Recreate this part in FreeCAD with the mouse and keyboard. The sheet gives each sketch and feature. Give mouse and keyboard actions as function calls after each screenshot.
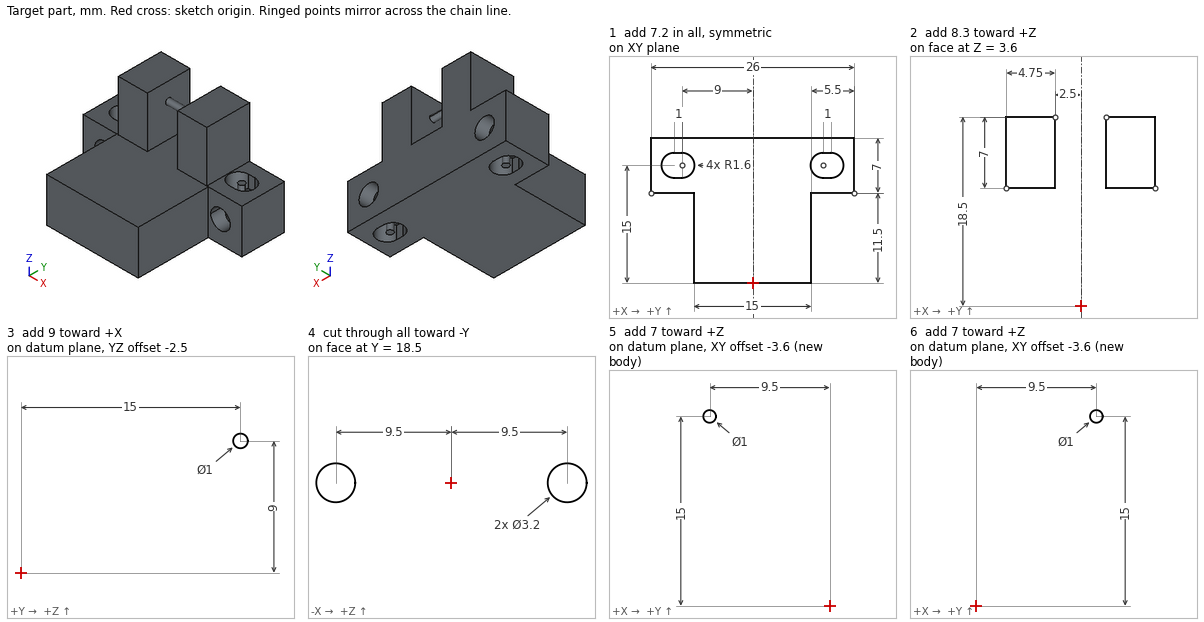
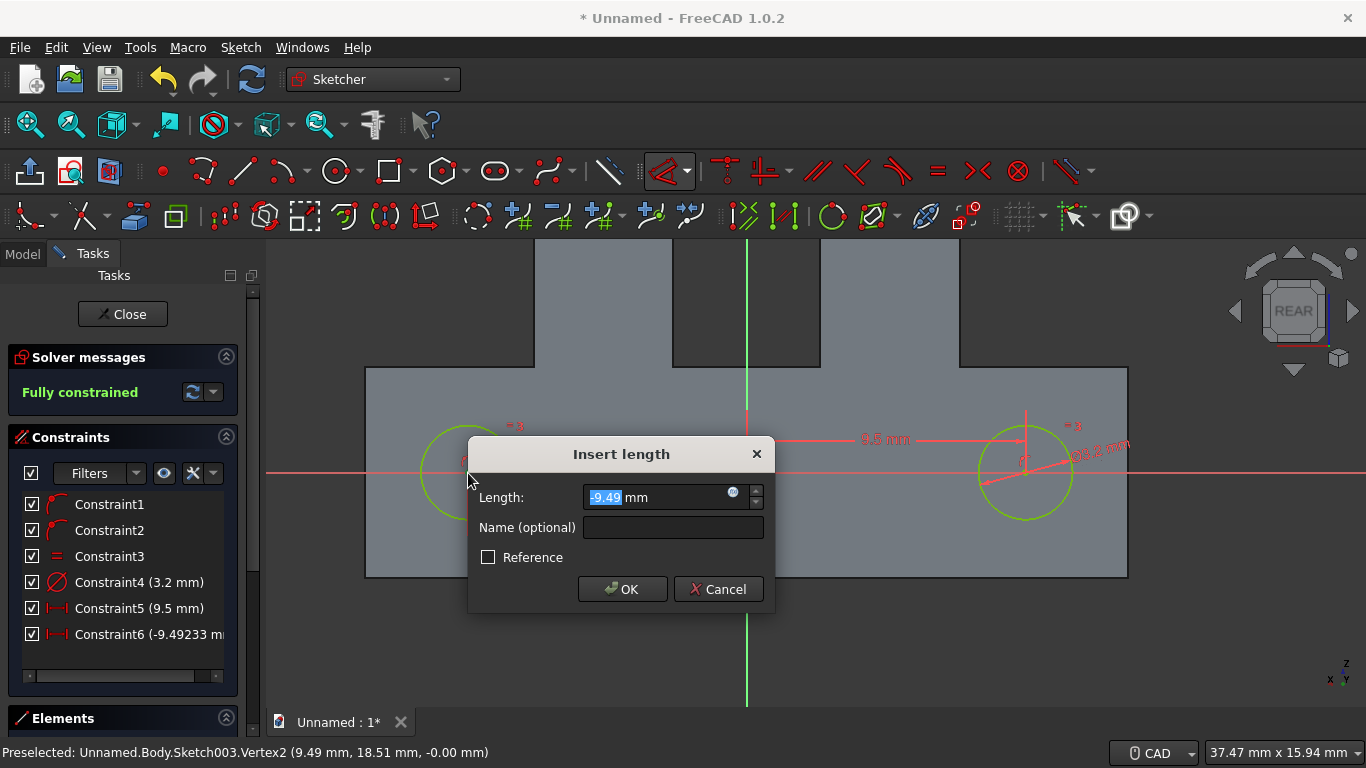
text(-9.5)
key(Return)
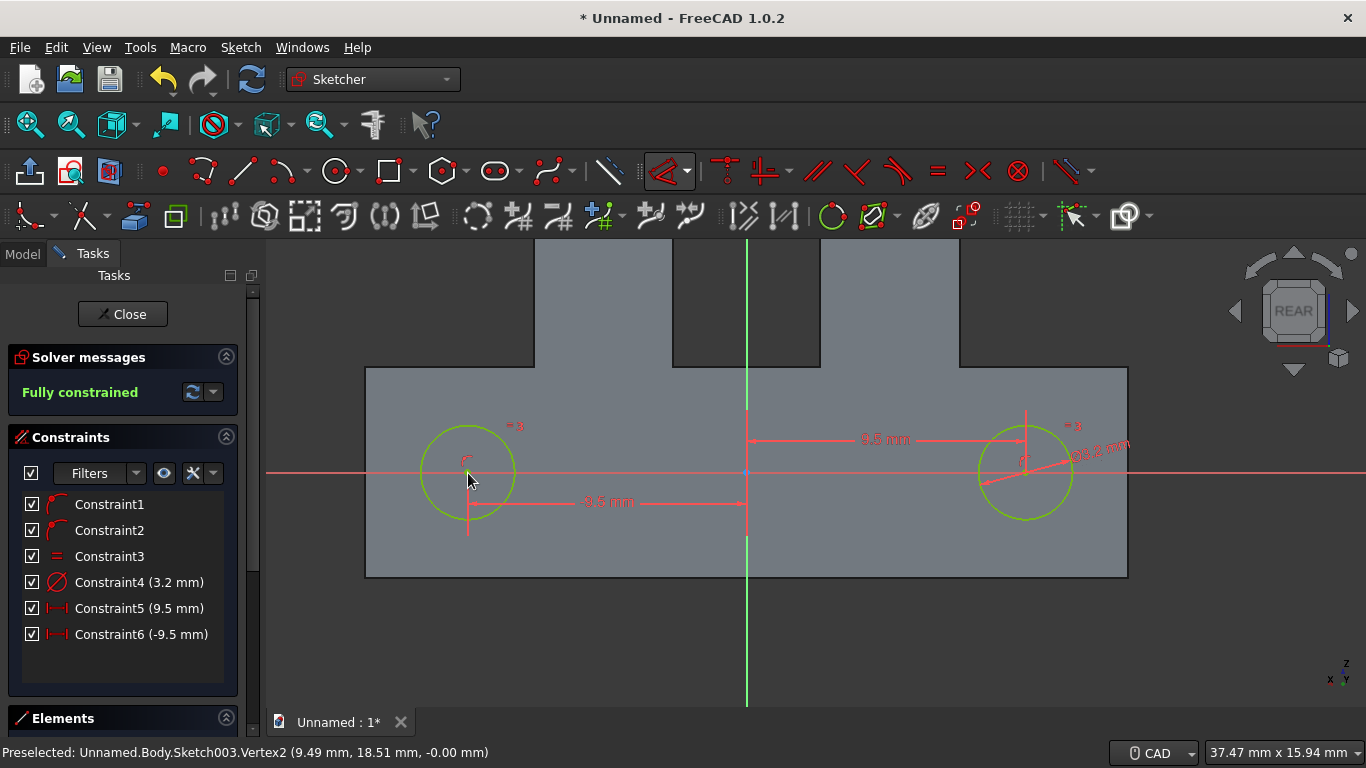
click(123, 314)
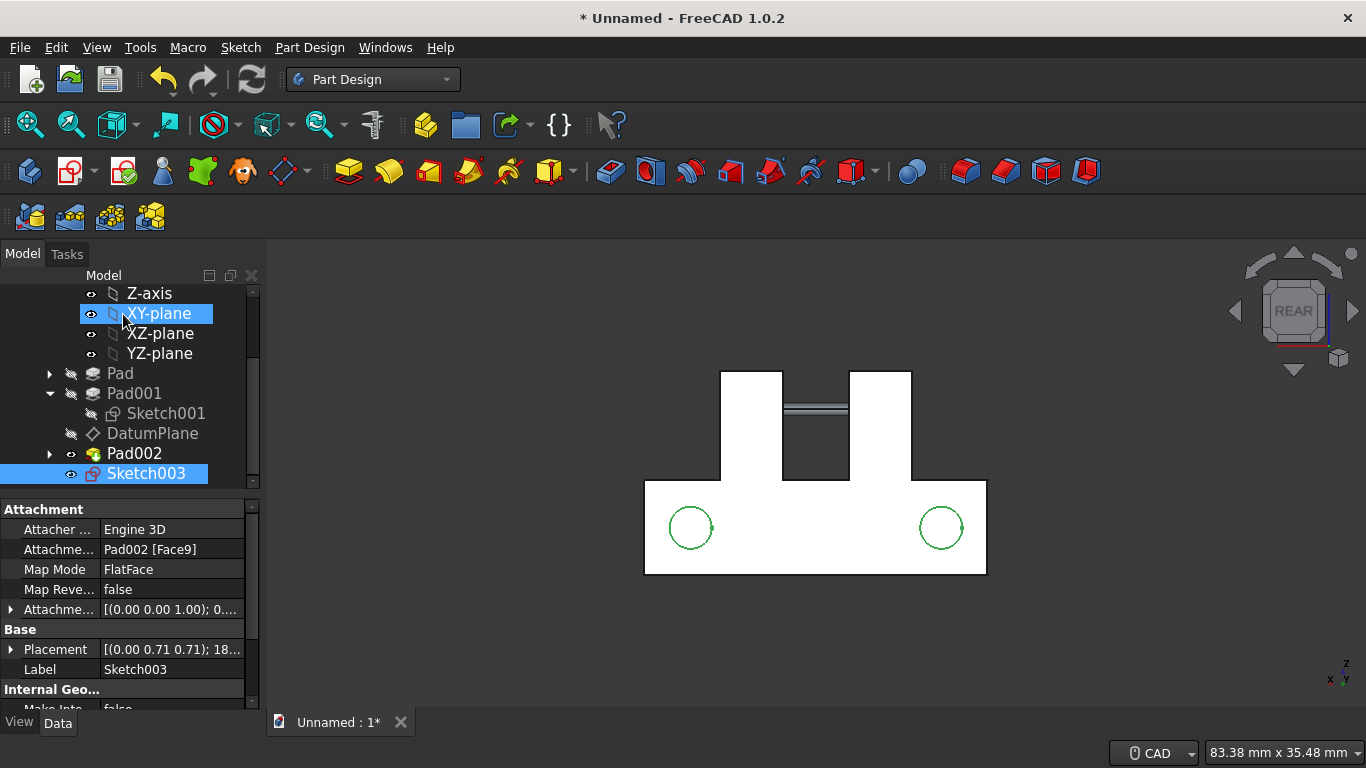
click(612, 172)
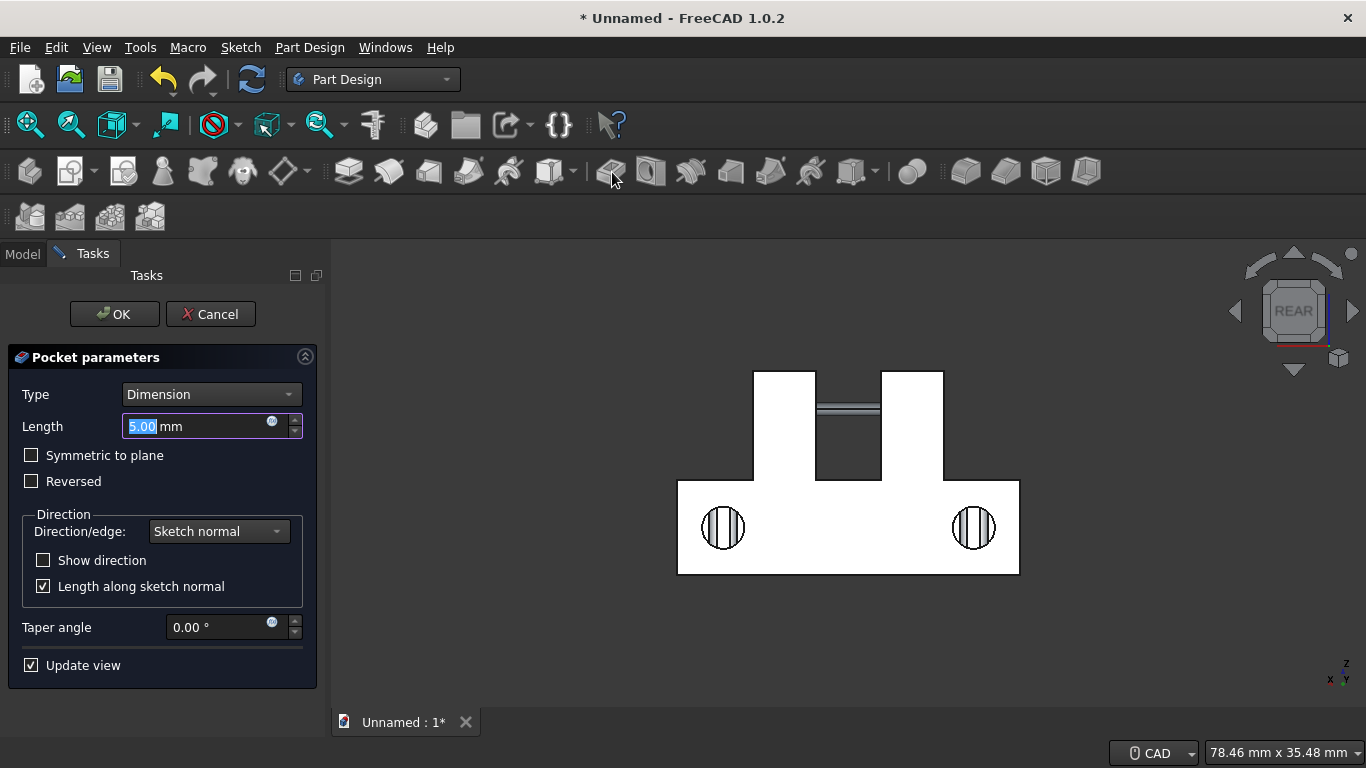
click(212, 394)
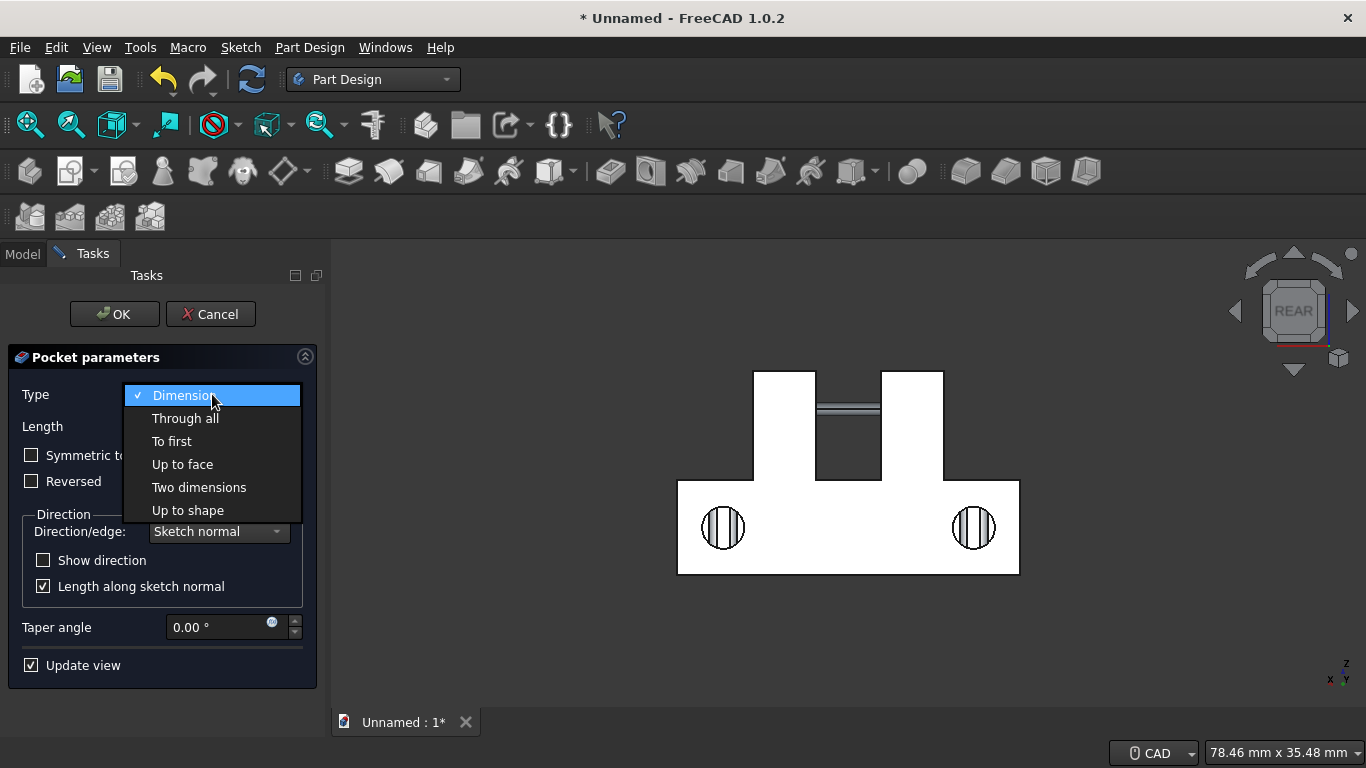
click(212, 418)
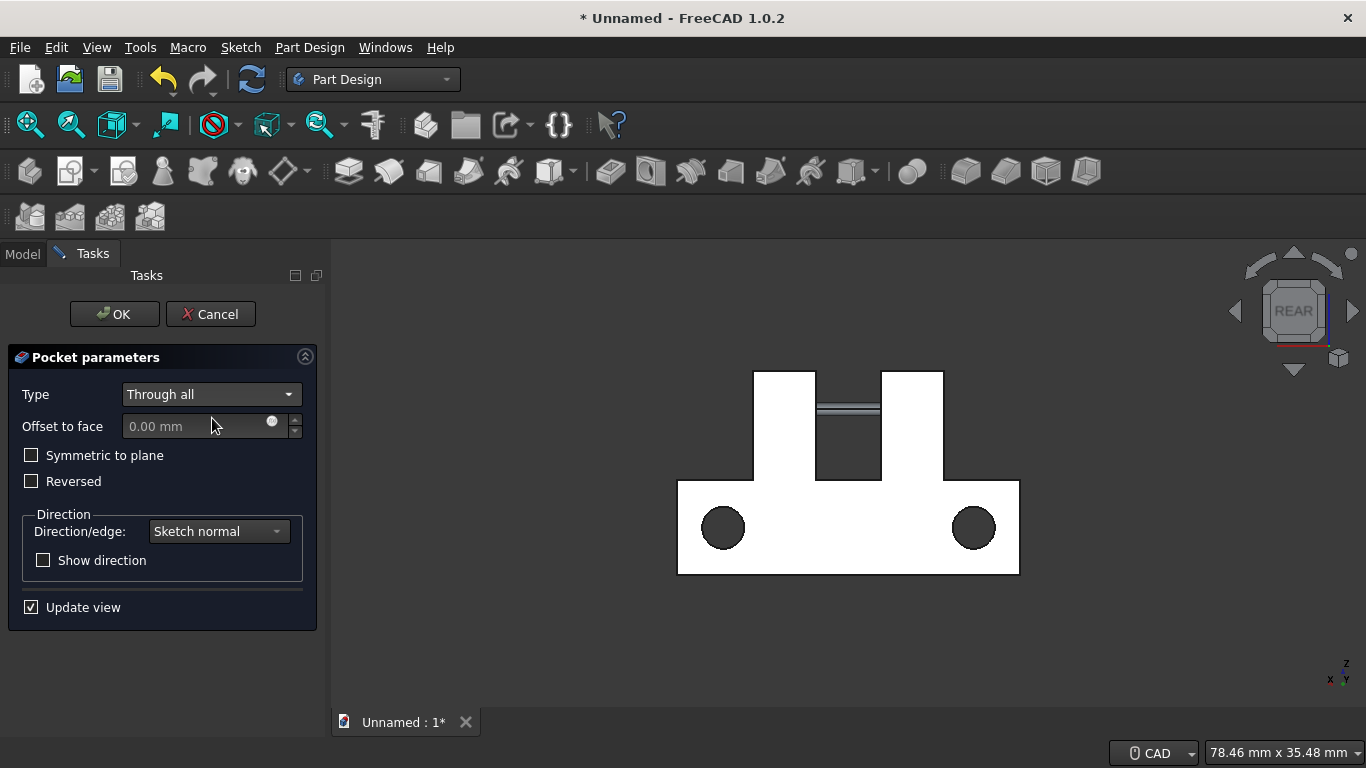
click(115, 314)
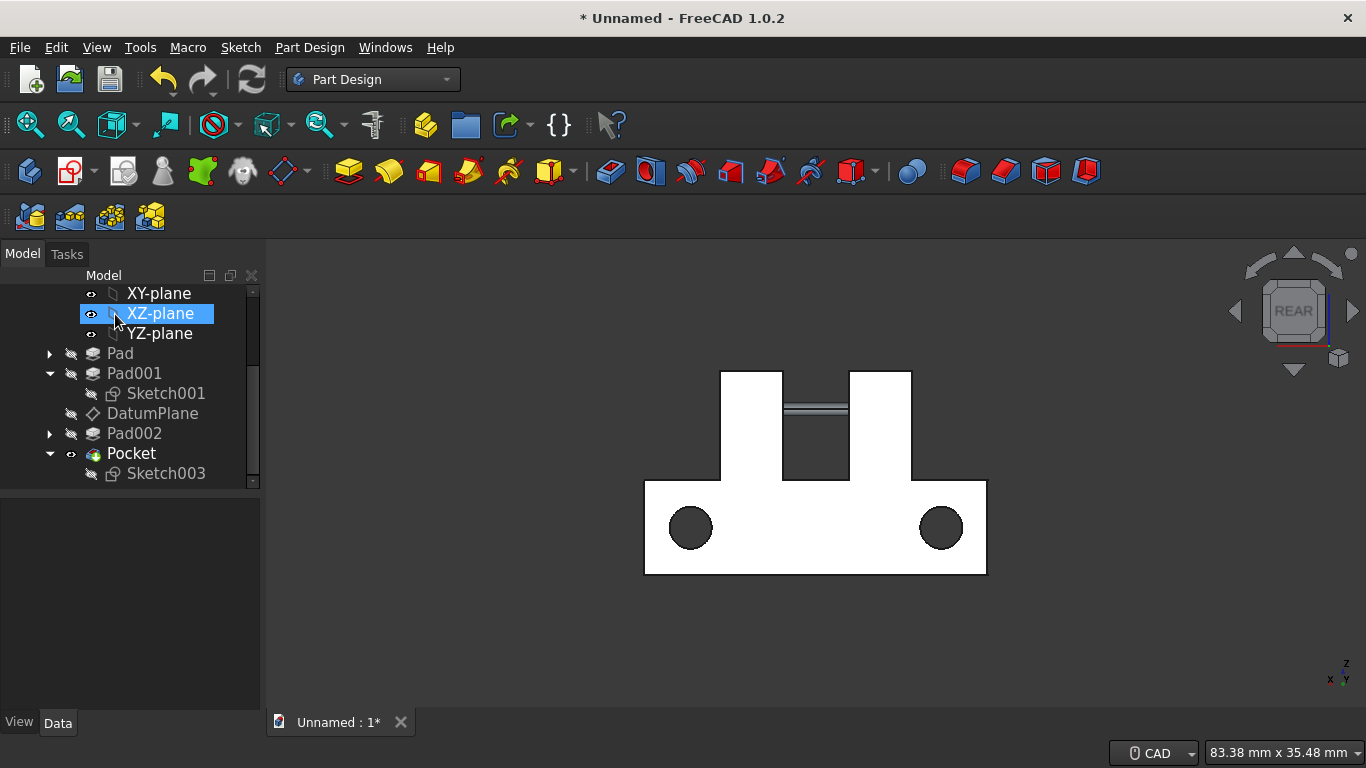
key(v)
key(f)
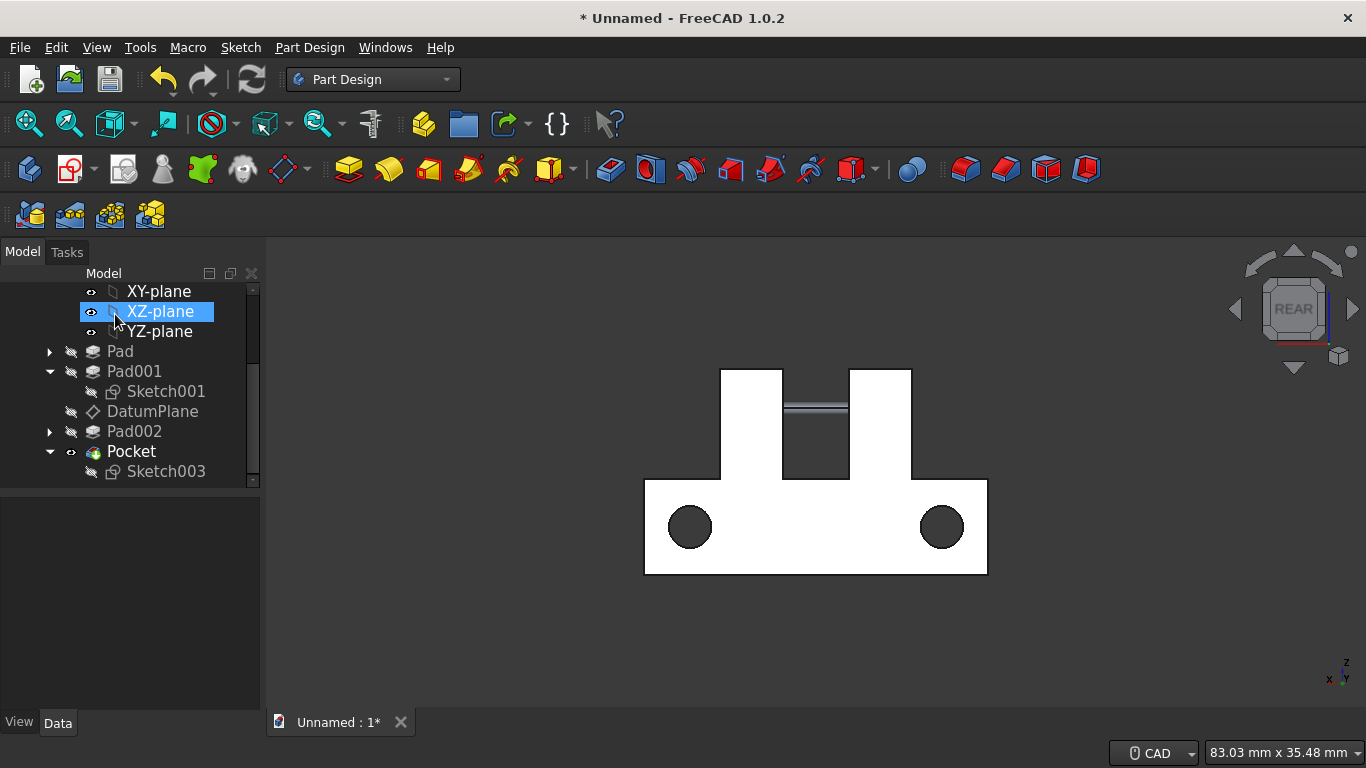
click(30, 170)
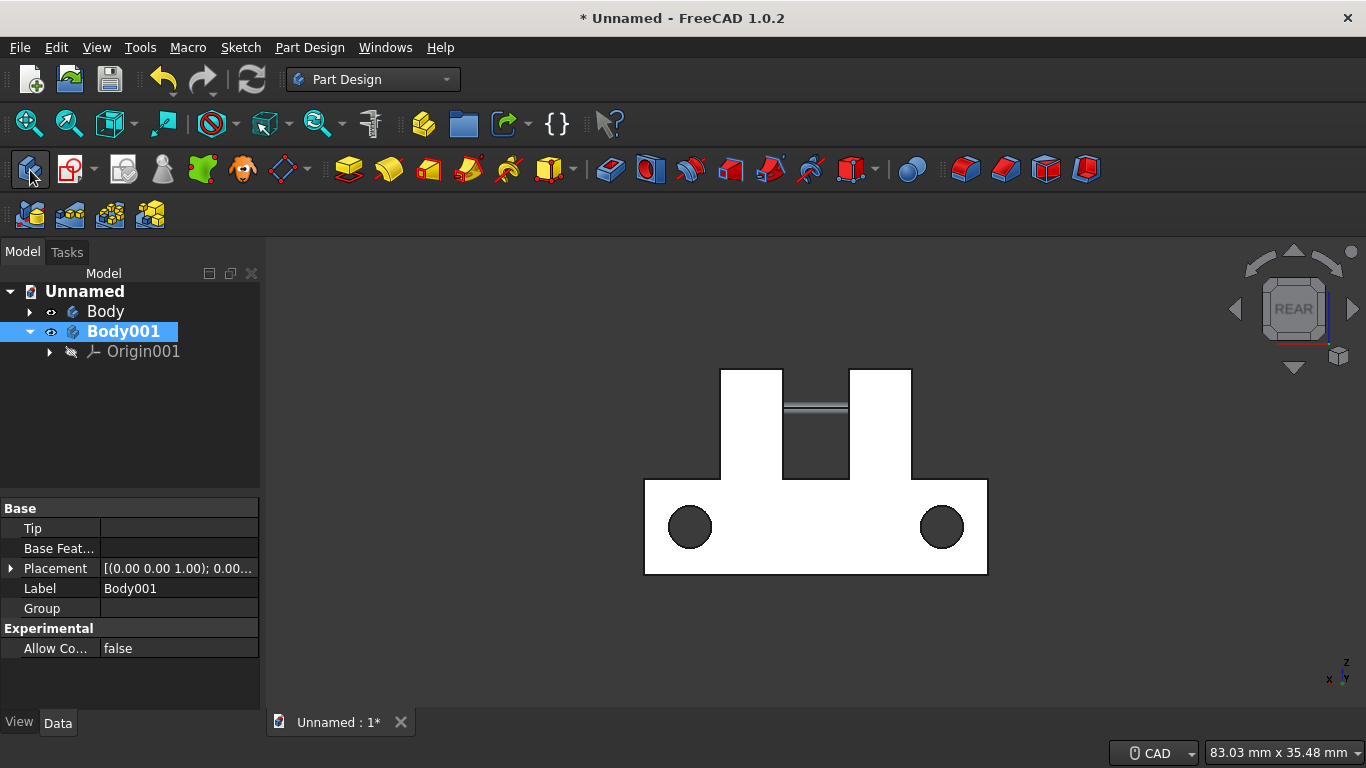
click(50, 352)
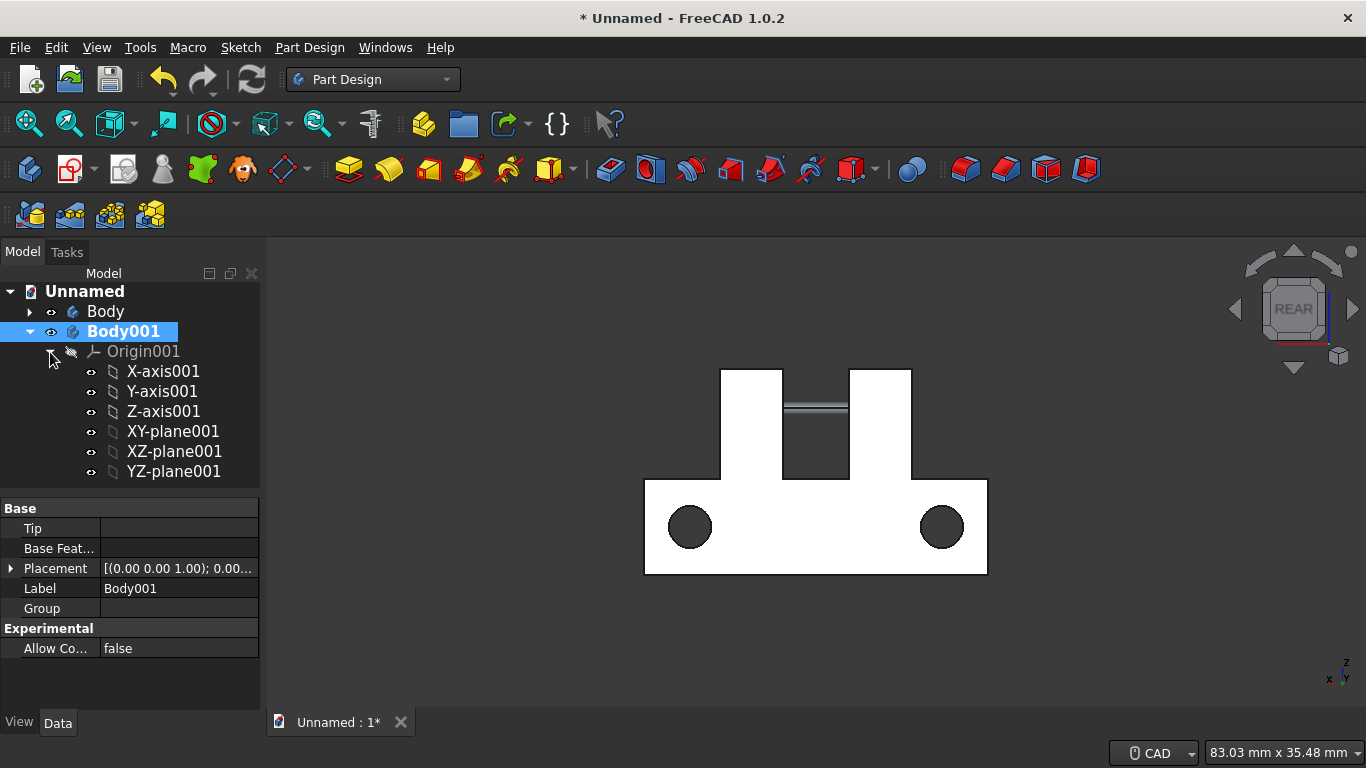
click(136, 432)